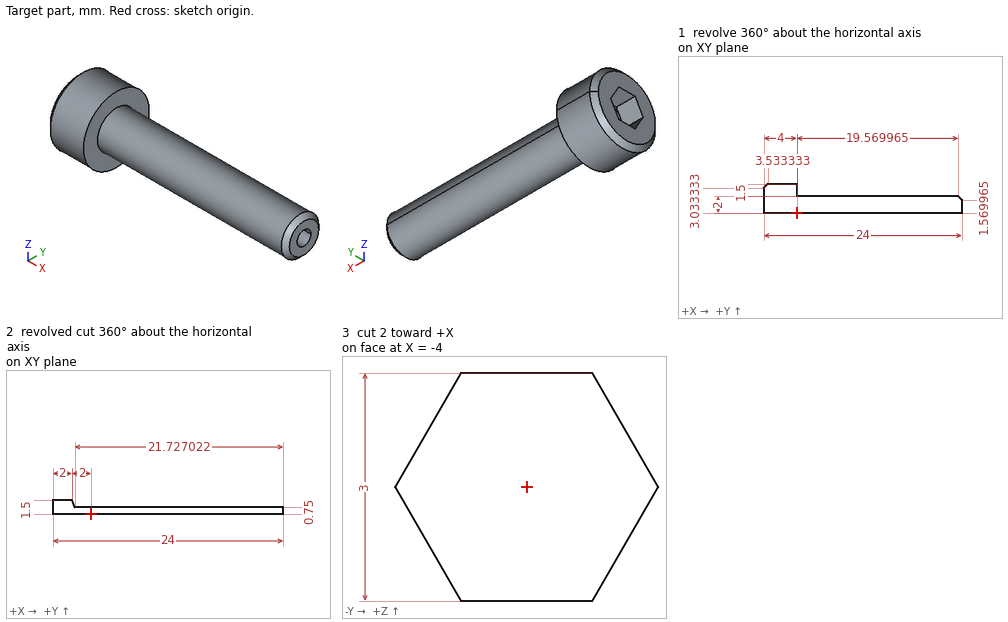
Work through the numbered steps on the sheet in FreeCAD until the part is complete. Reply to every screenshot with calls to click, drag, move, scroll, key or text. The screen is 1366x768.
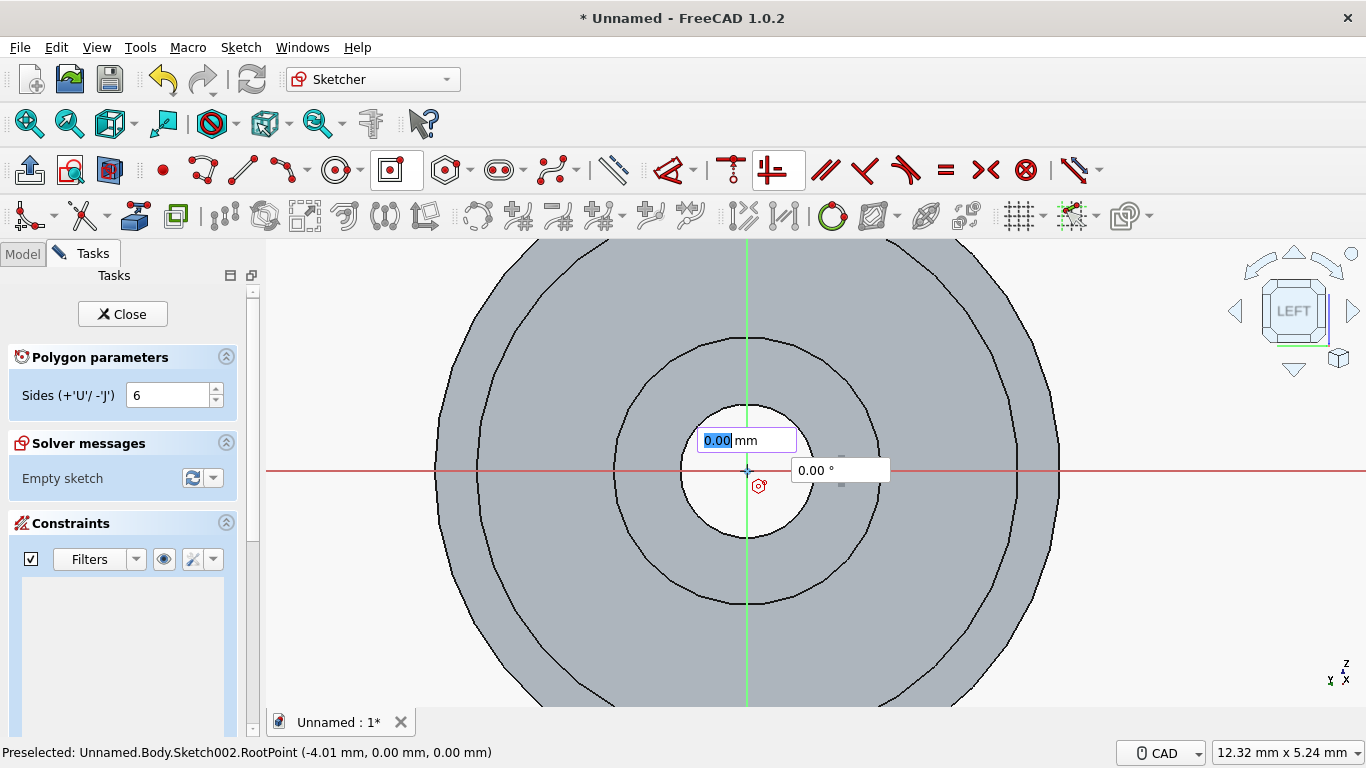
click(902, 471)
key(Escape)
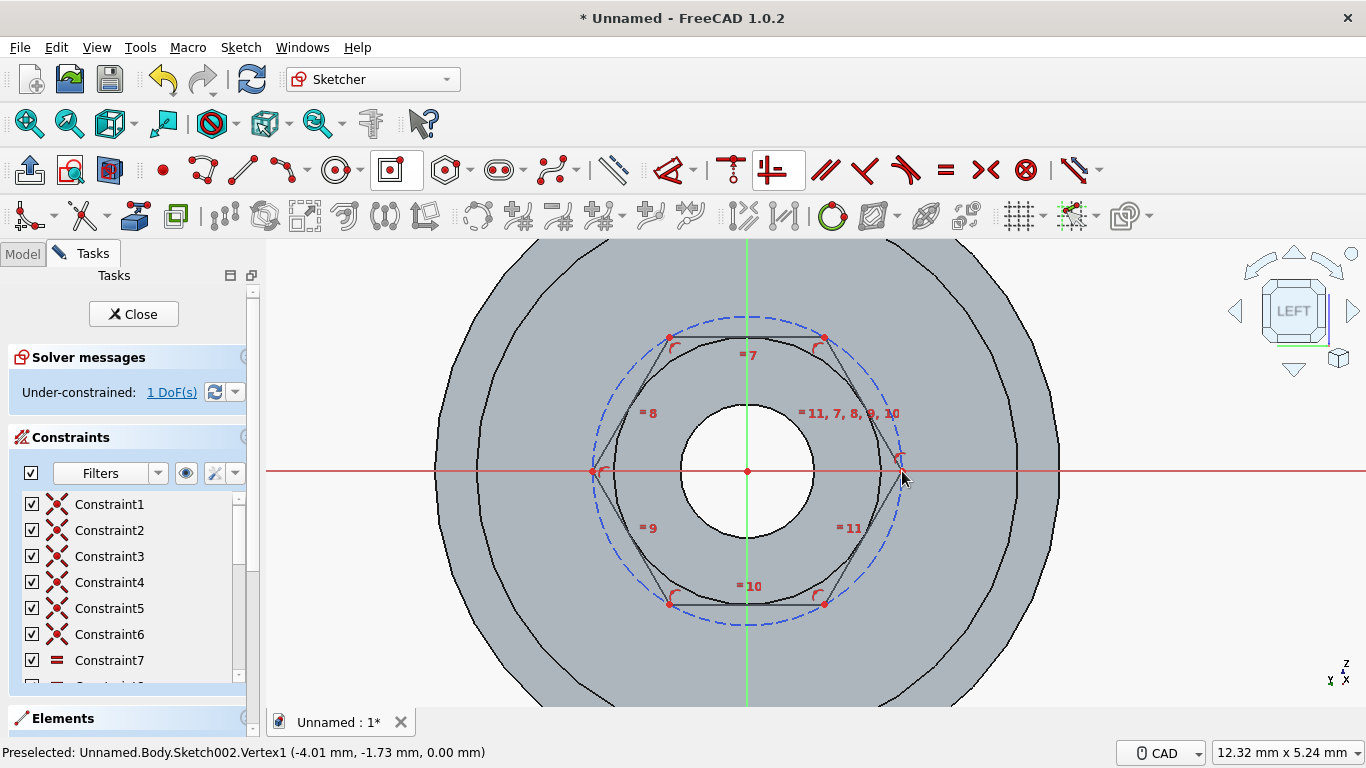
click(668, 170)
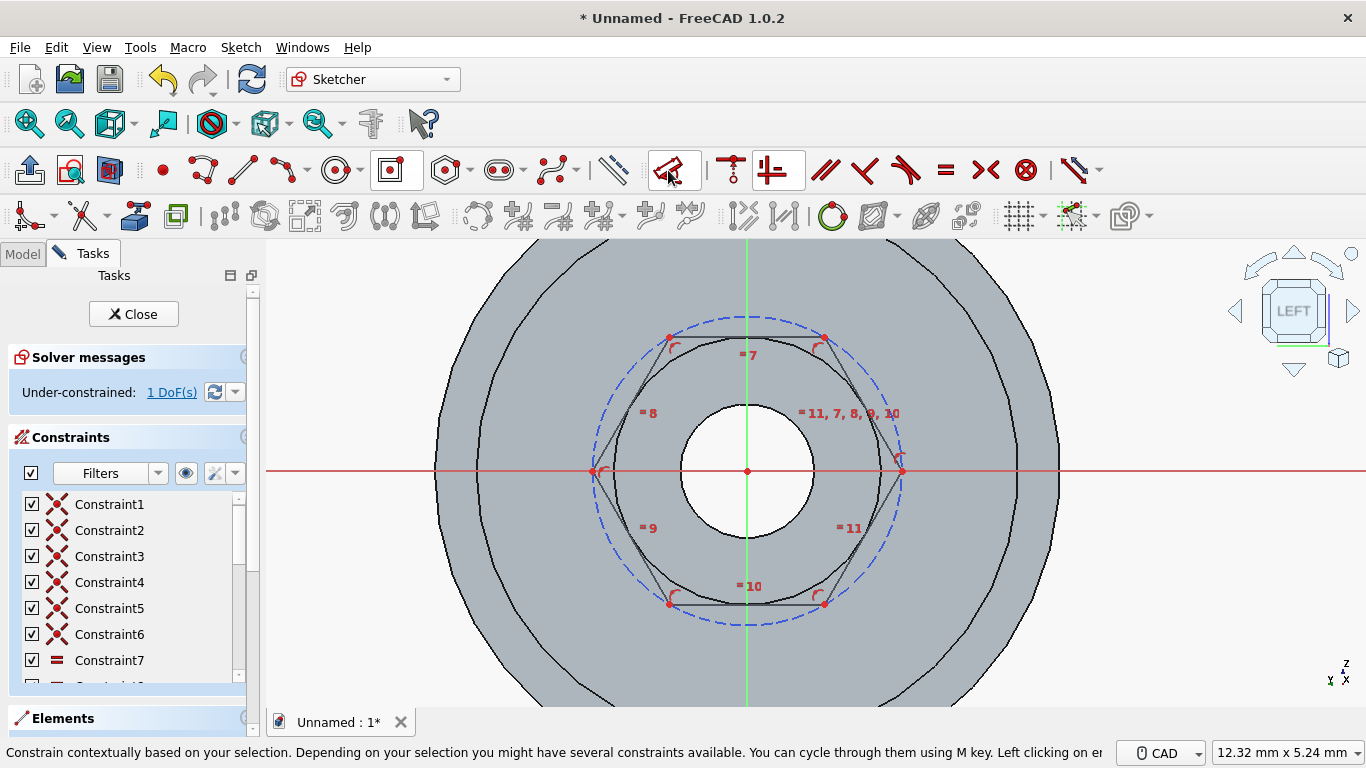
click(670, 605)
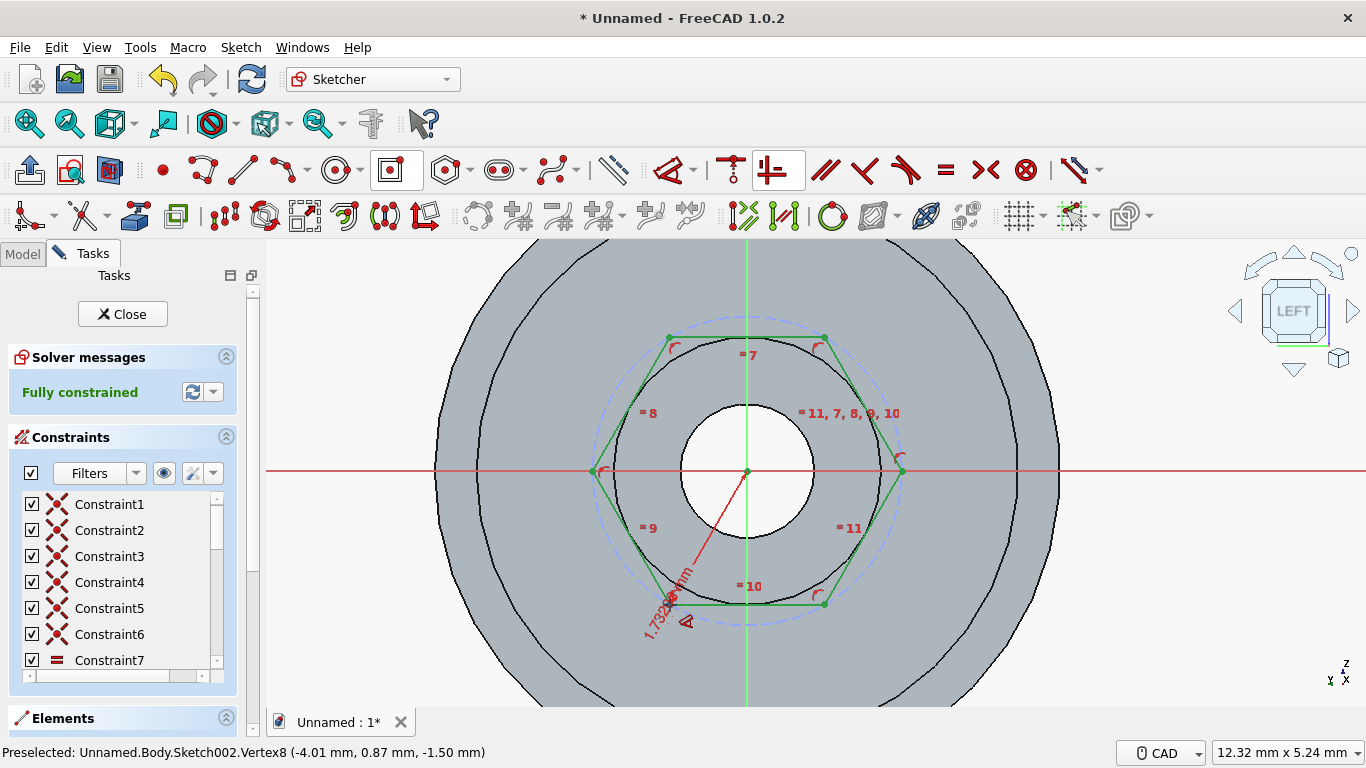
click(825, 337)
click(907, 409)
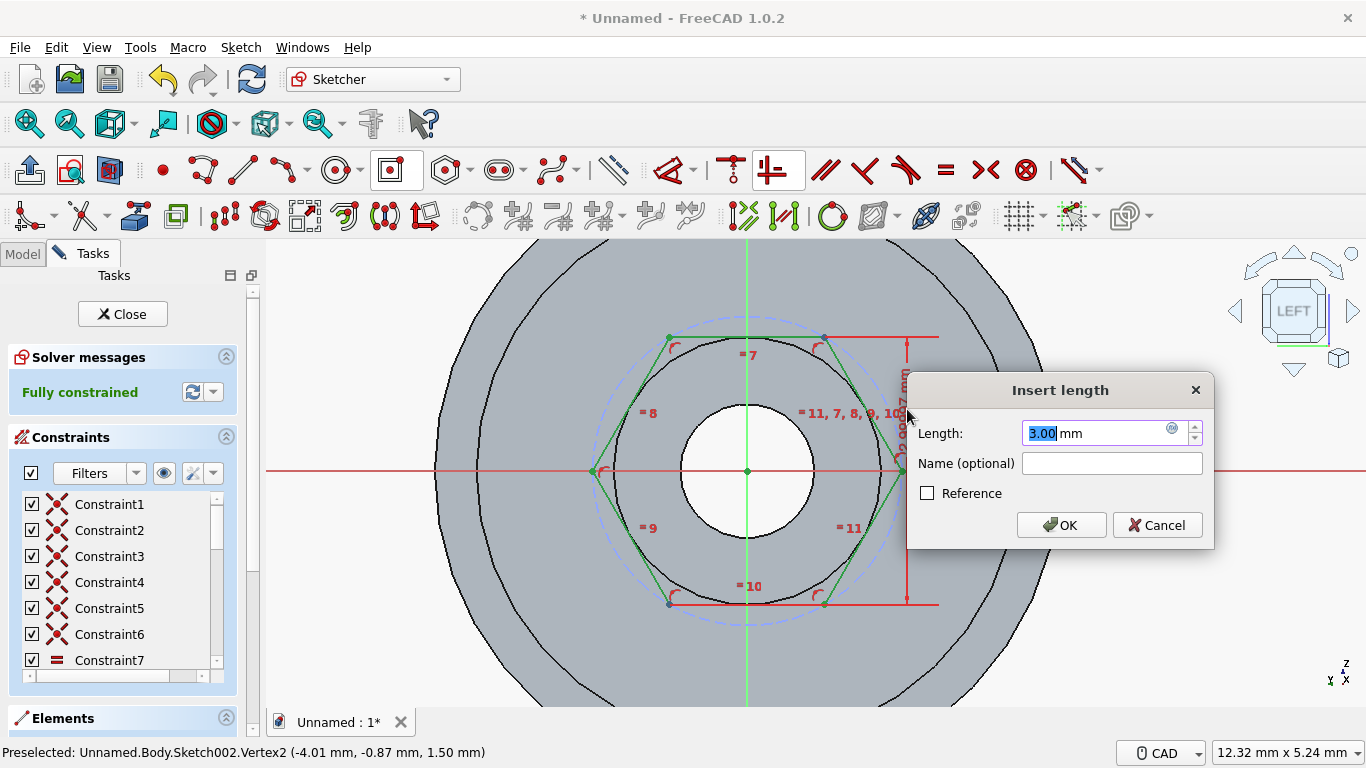
text(3)
key(Return)
key(Escape)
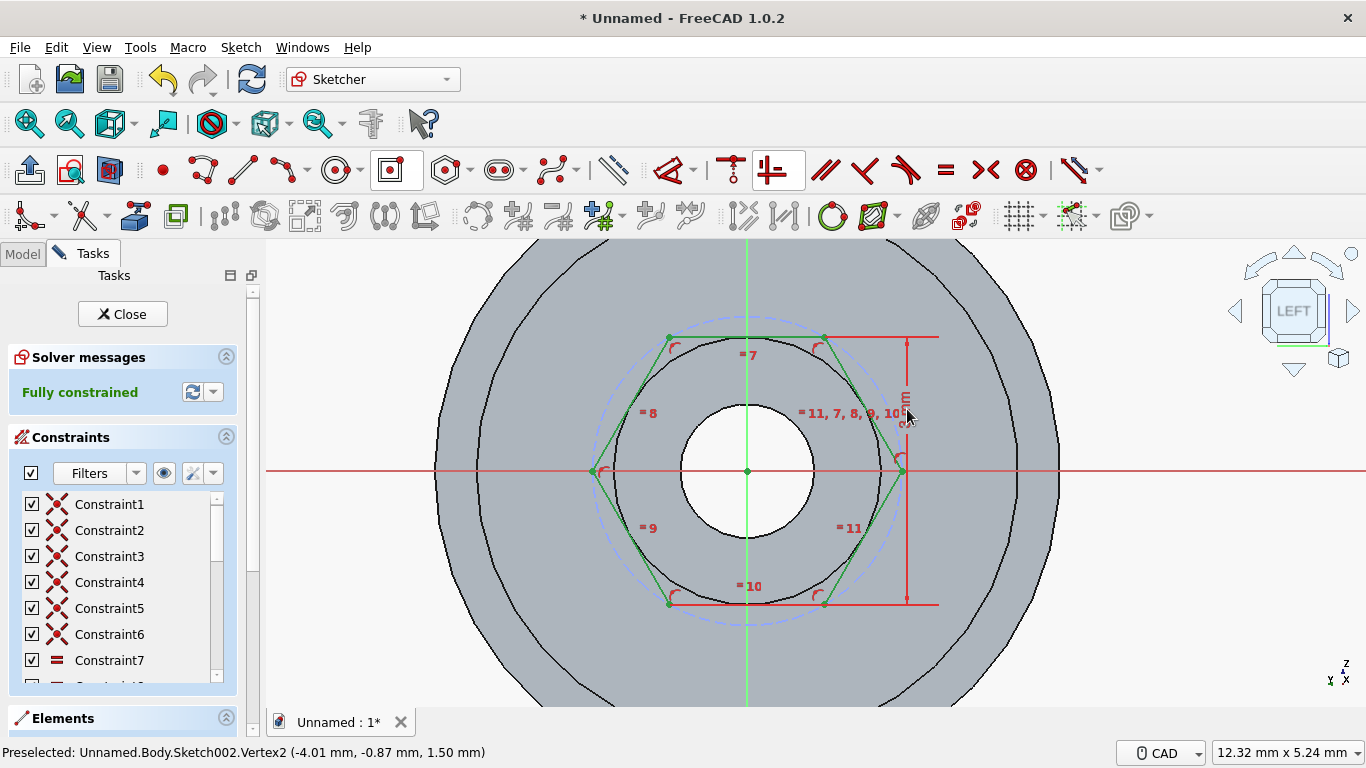
click(123, 314)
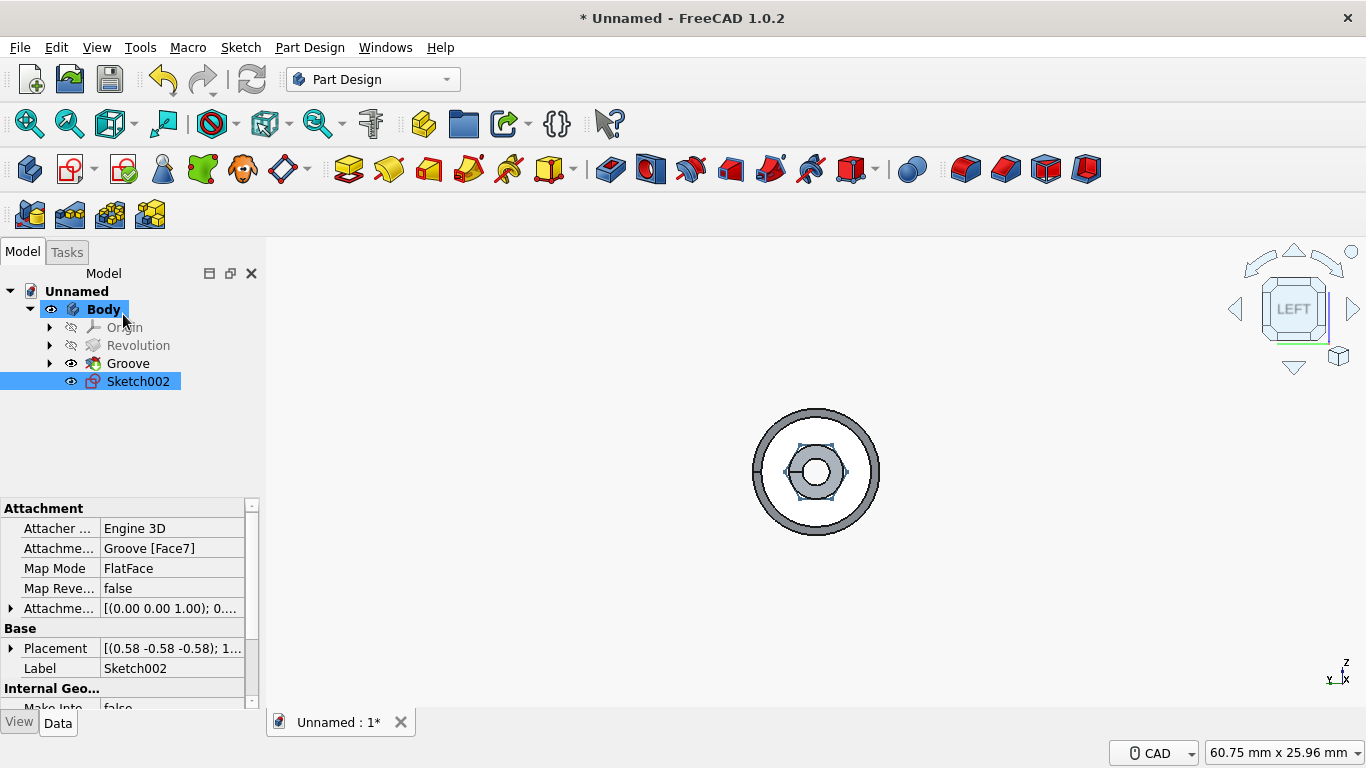
click(612, 170)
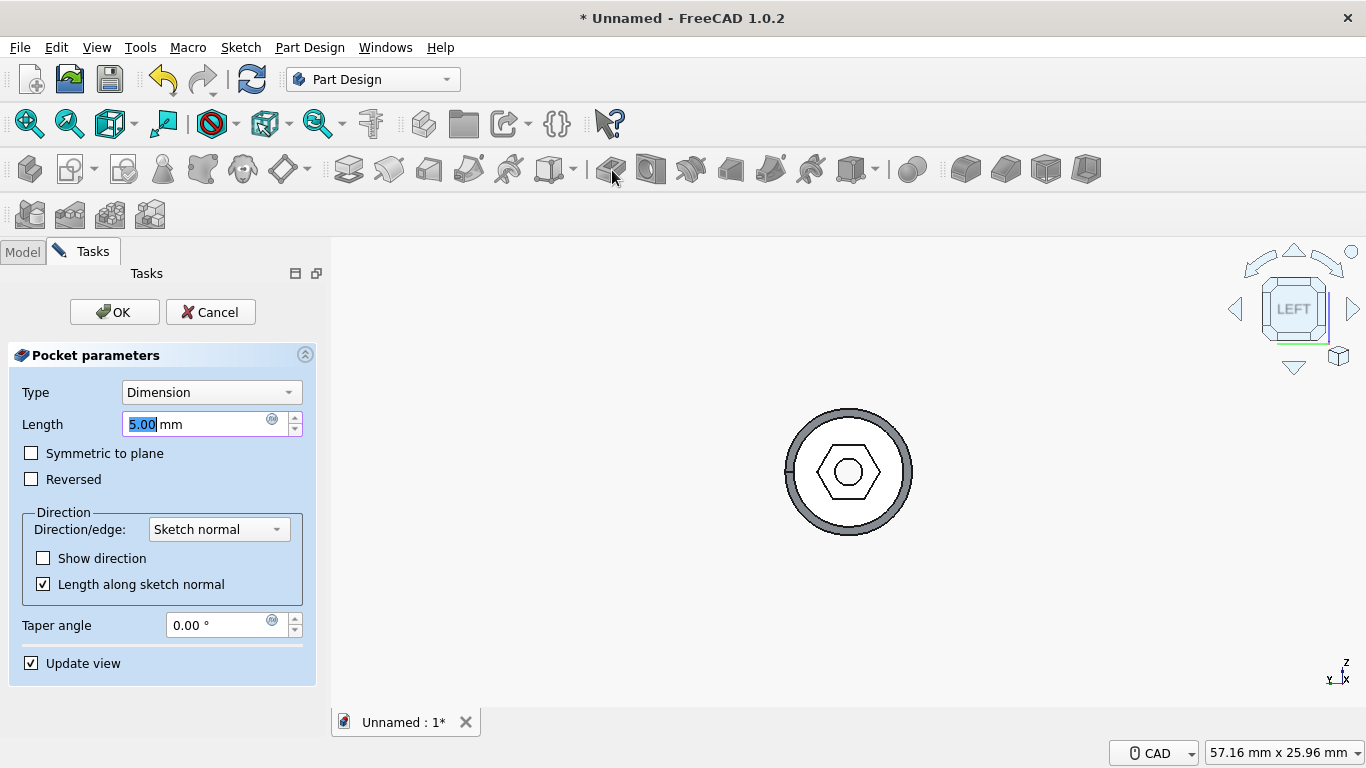
text(2)
key(Tab)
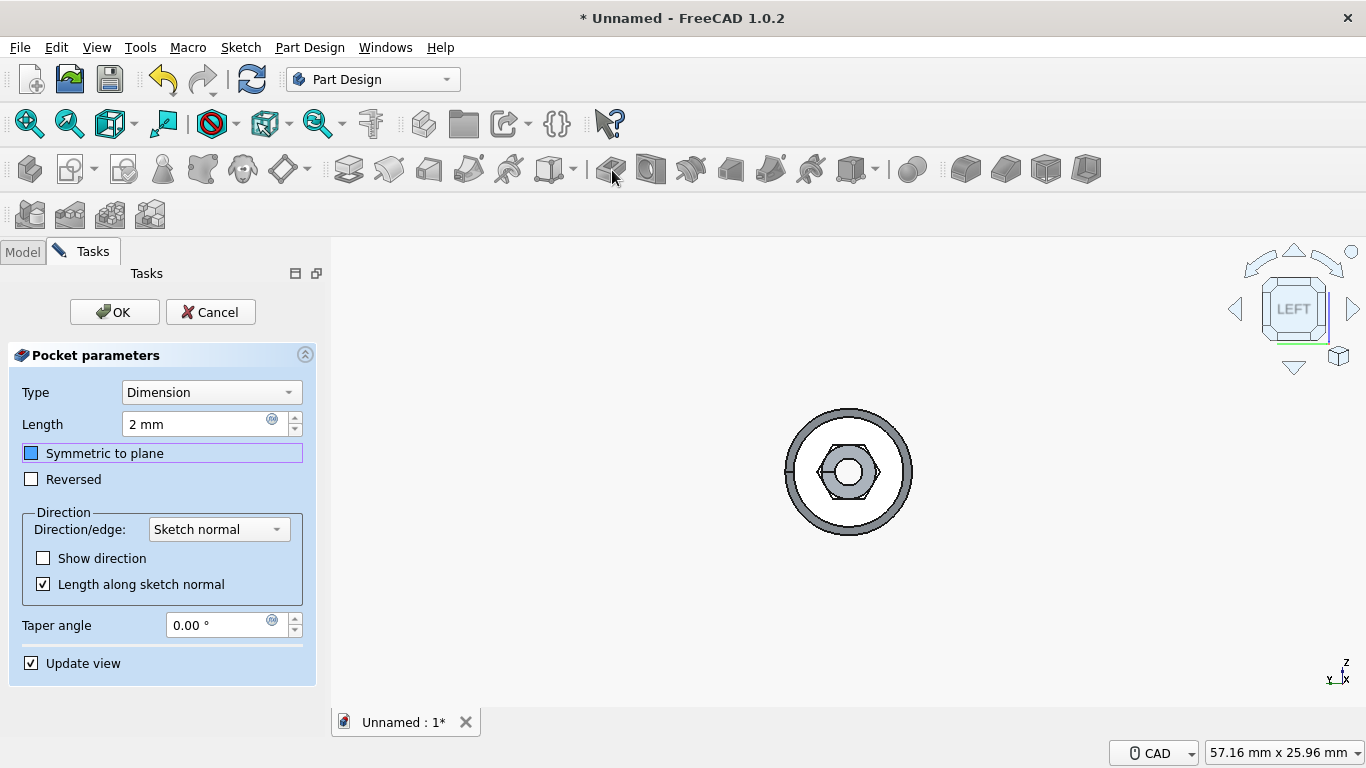
click(115, 312)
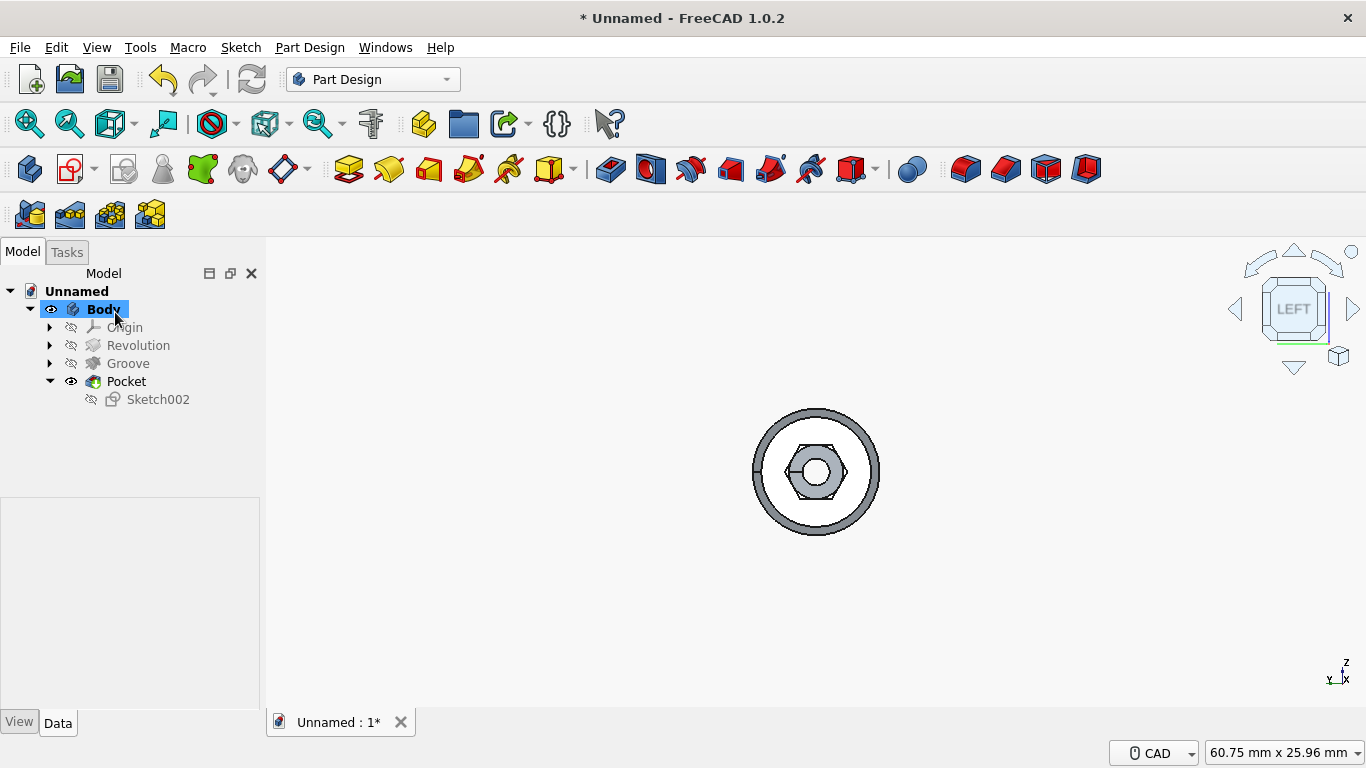
key(0)